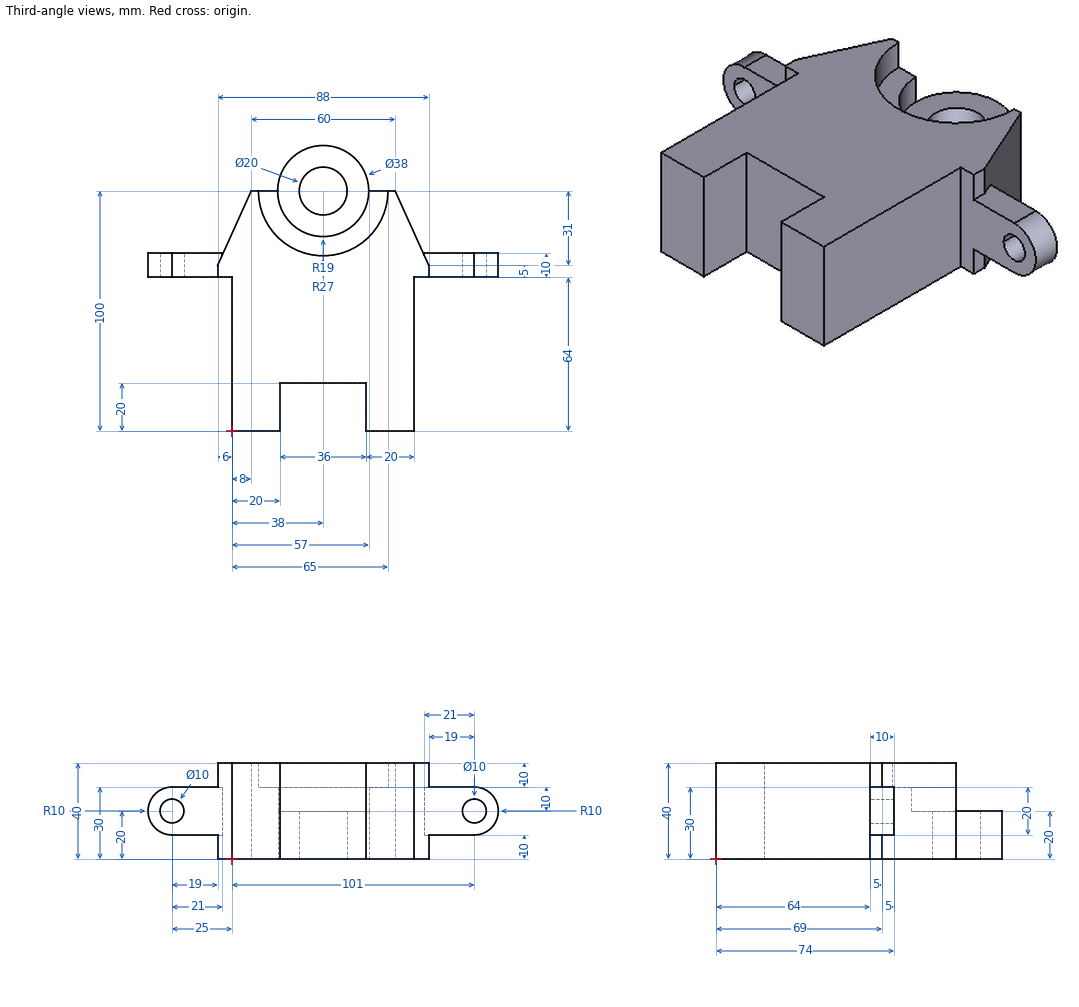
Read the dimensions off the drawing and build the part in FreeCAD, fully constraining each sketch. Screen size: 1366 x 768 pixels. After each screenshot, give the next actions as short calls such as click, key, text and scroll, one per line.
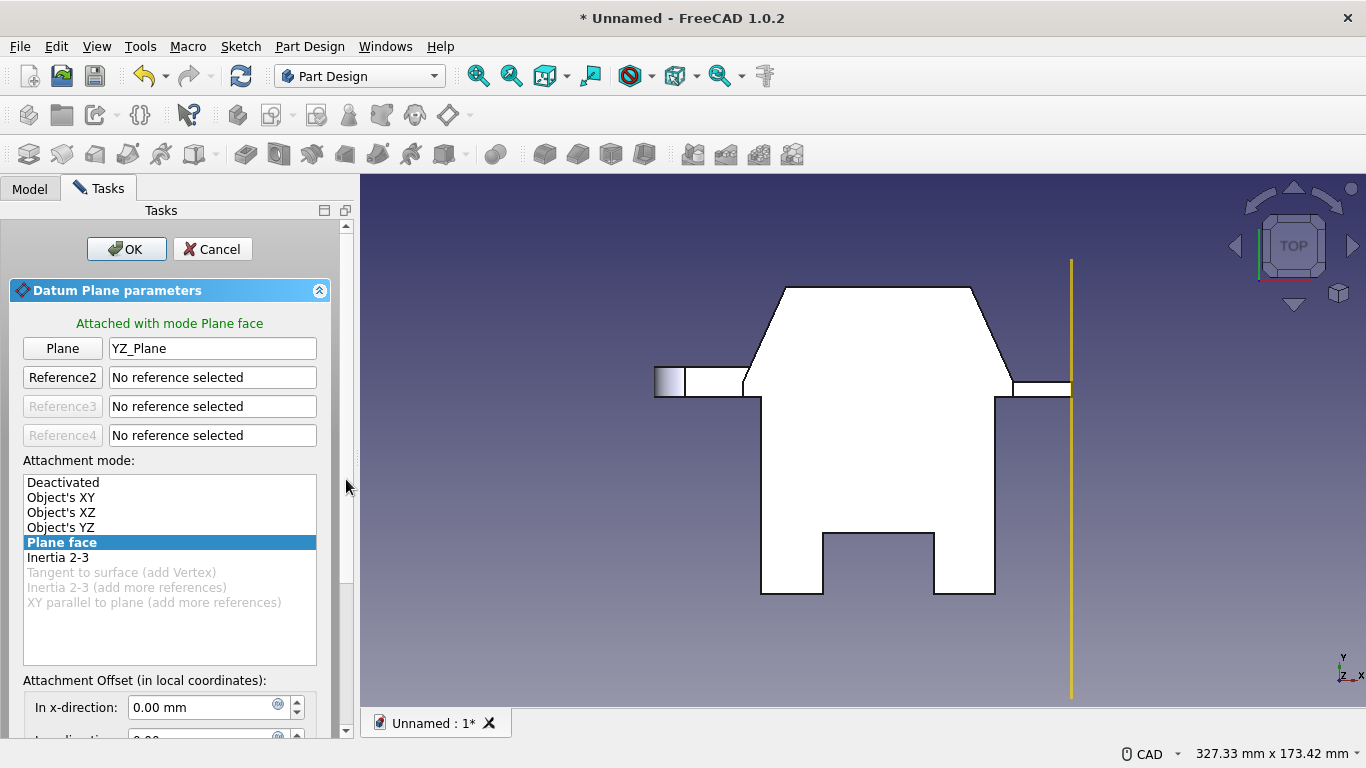
click(127, 249)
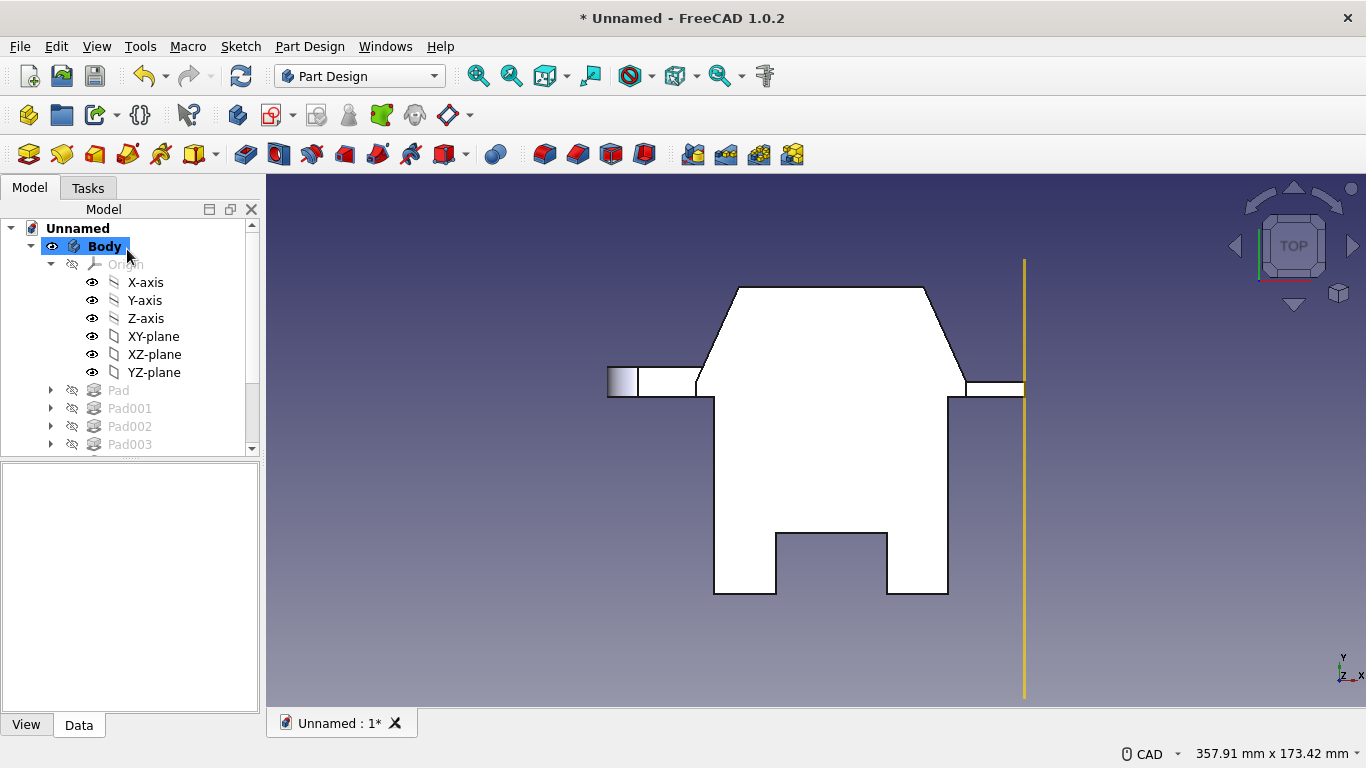
scroll(101, 332, down, 3)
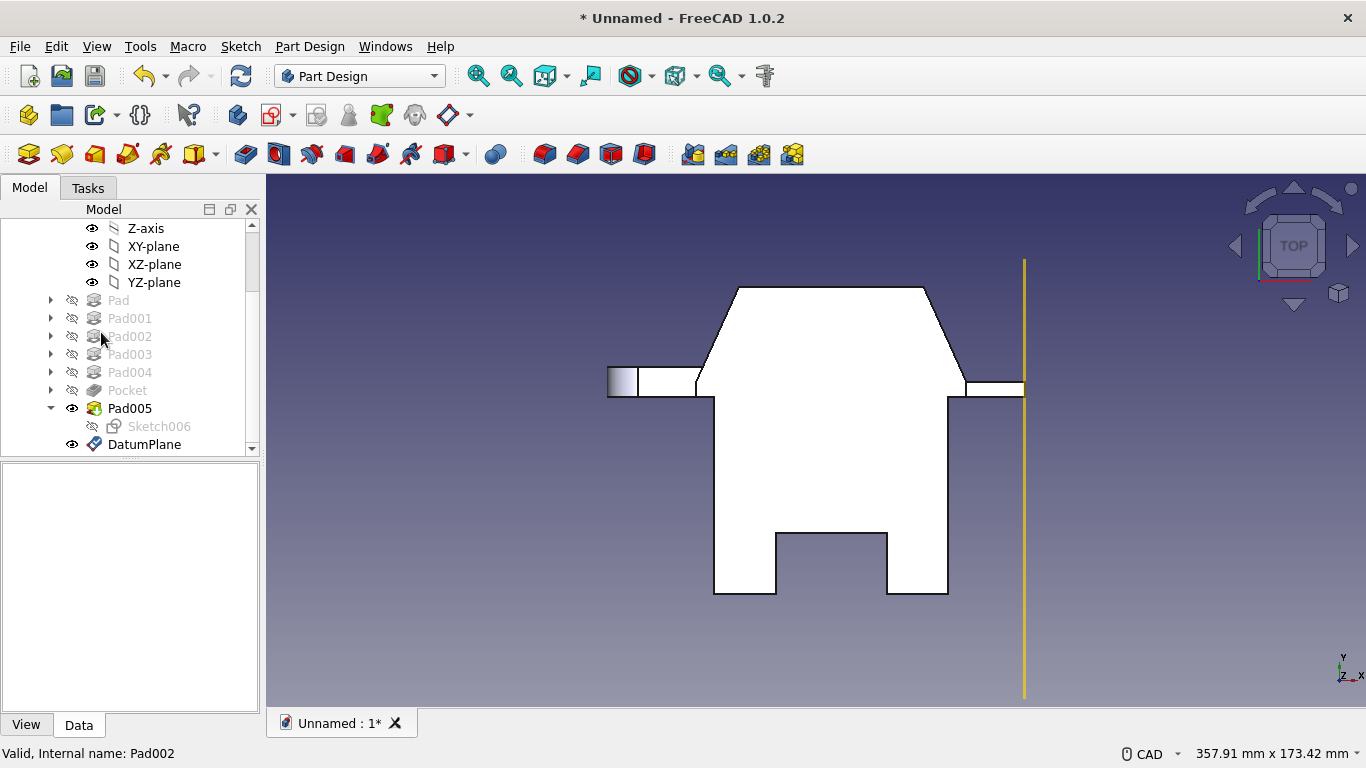
click(117, 444)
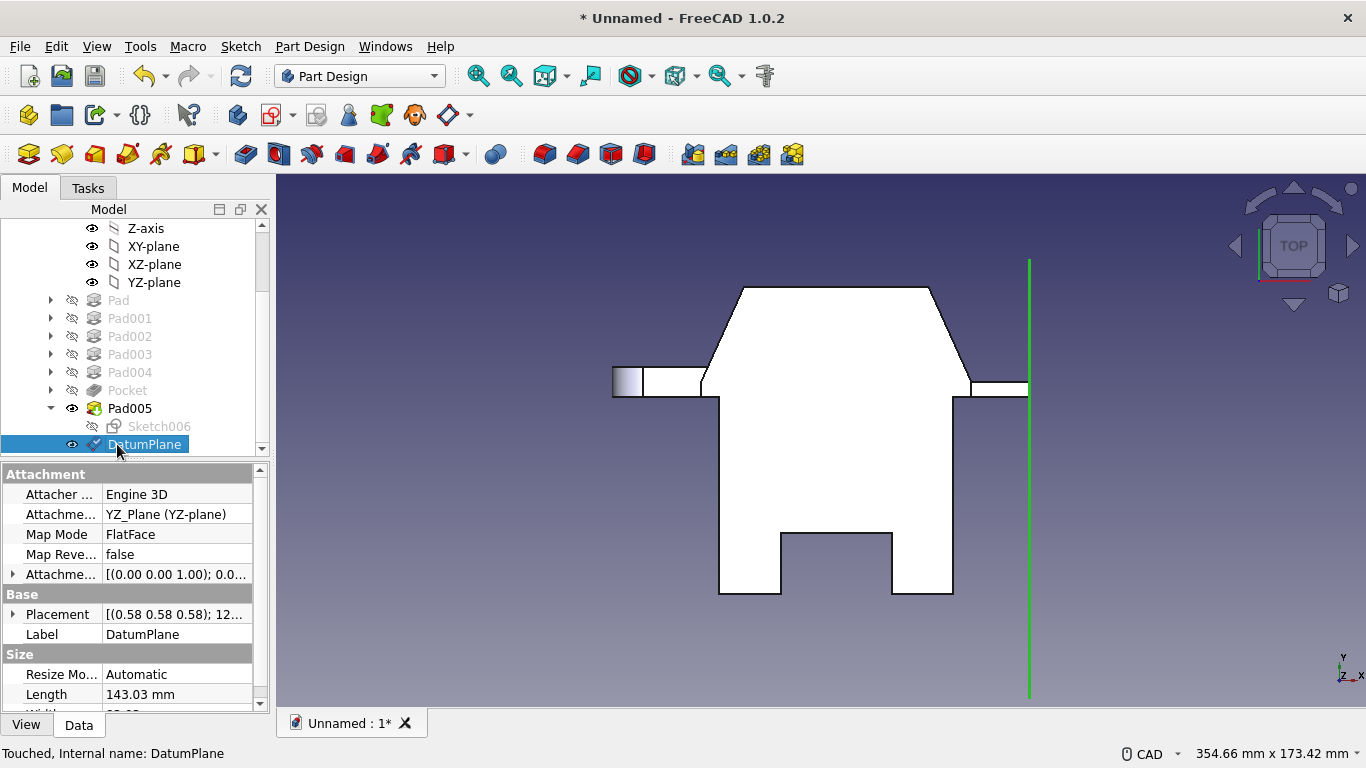
click(270, 116)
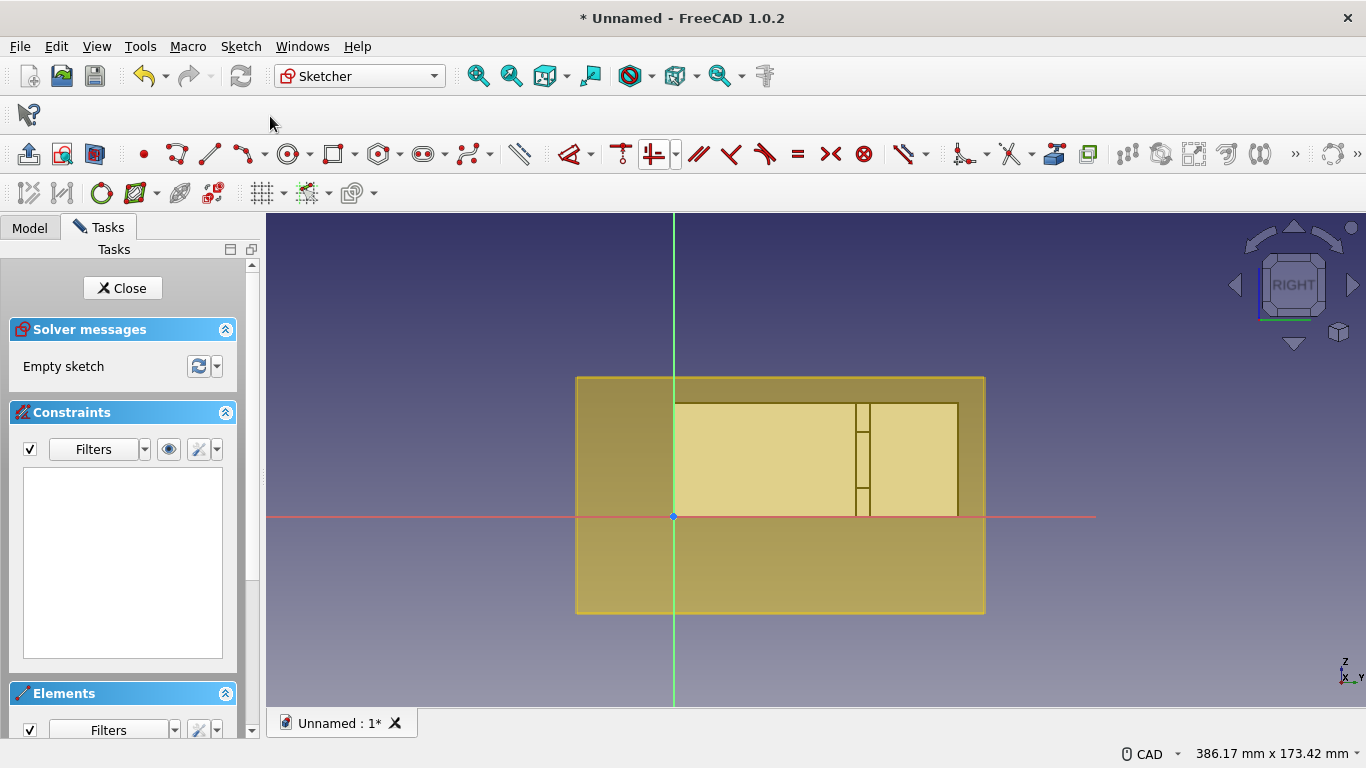
scroll(910, 460, up, 8)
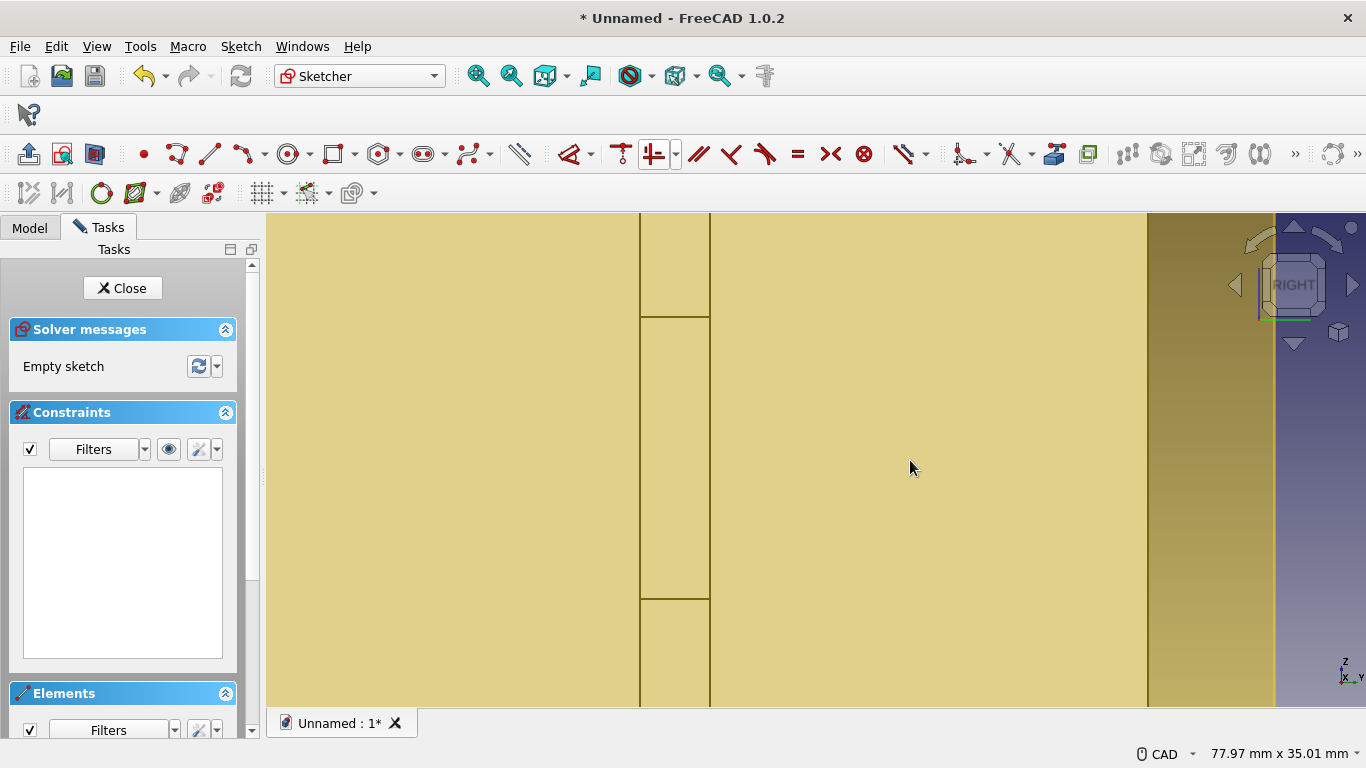
click(332, 154)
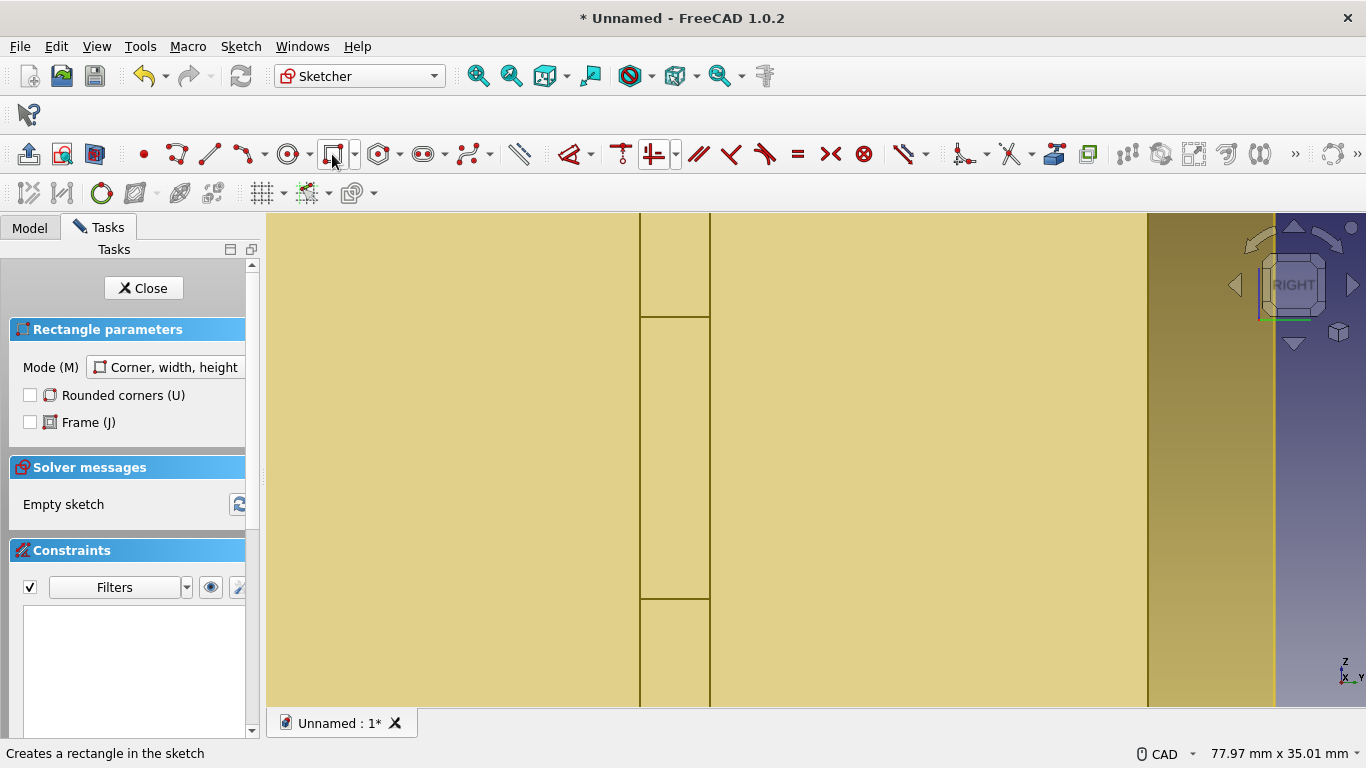
click(710, 317)
click(781, 599)
key(Escape)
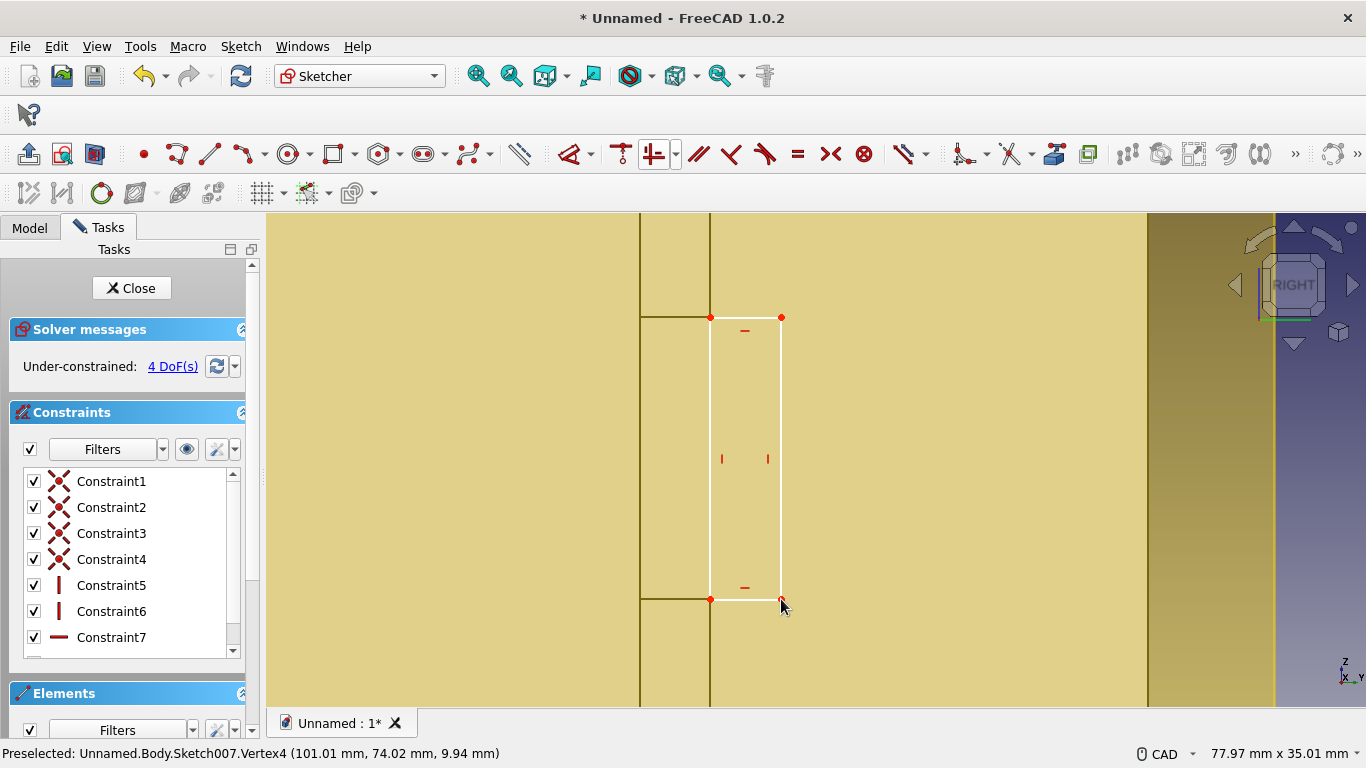
click(568, 154)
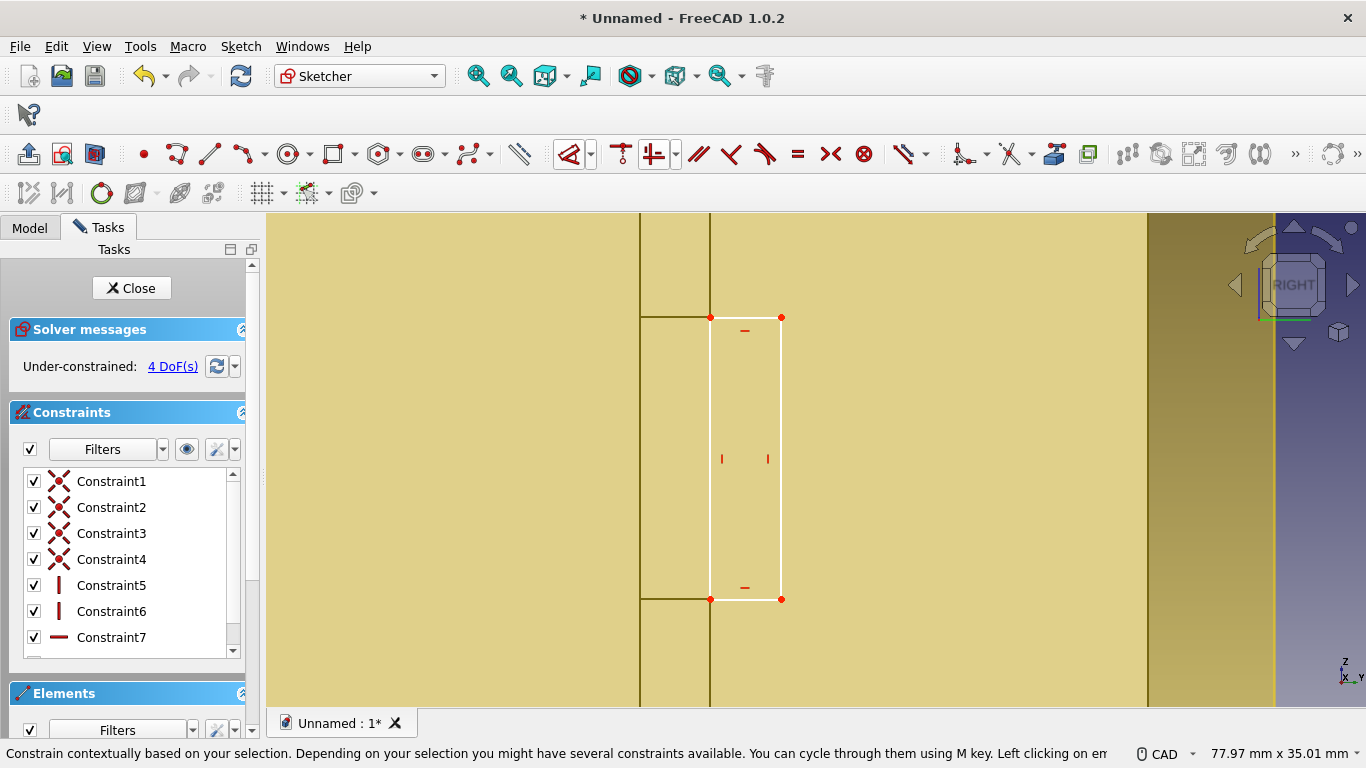
click(731, 600)
click(745, 634)